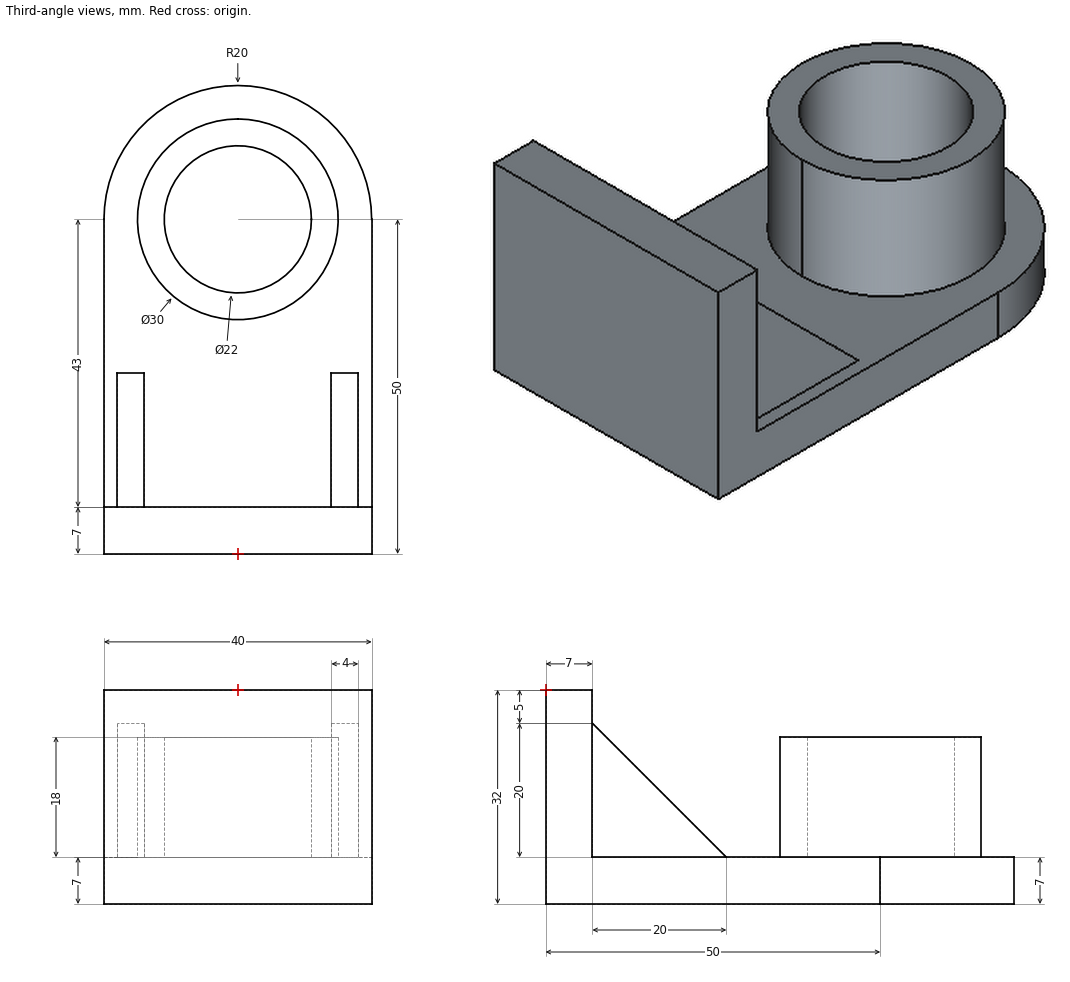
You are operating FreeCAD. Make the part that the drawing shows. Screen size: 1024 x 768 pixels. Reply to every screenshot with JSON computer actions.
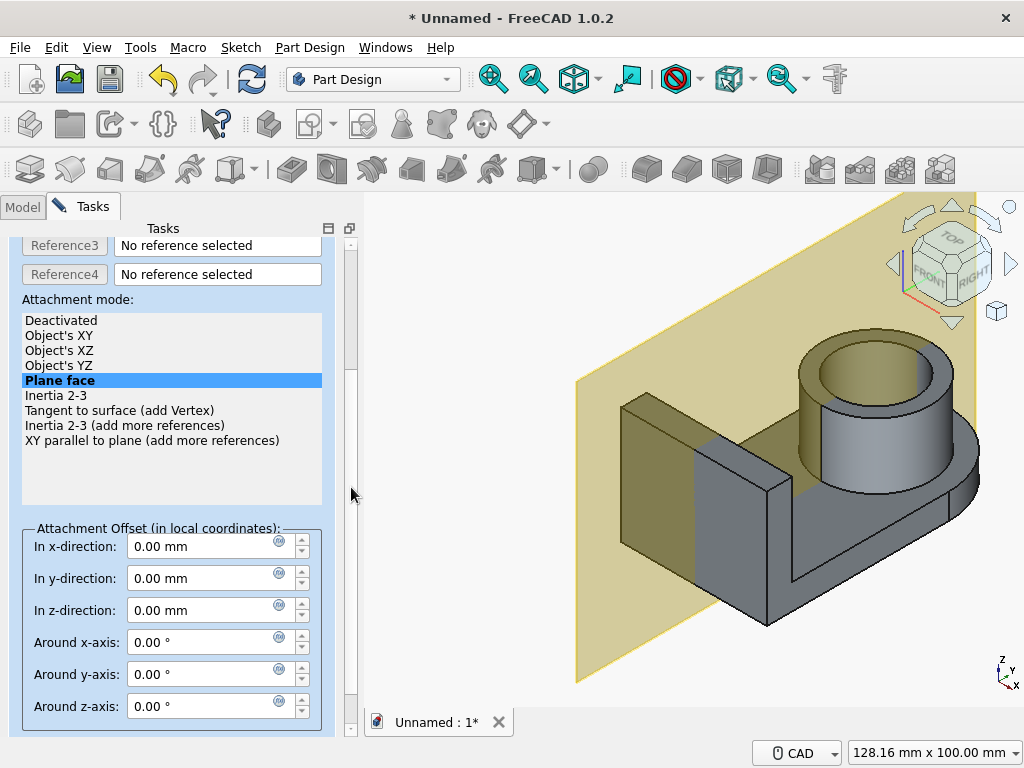
{"action": "triple_click", "coordinate": [210, 610]}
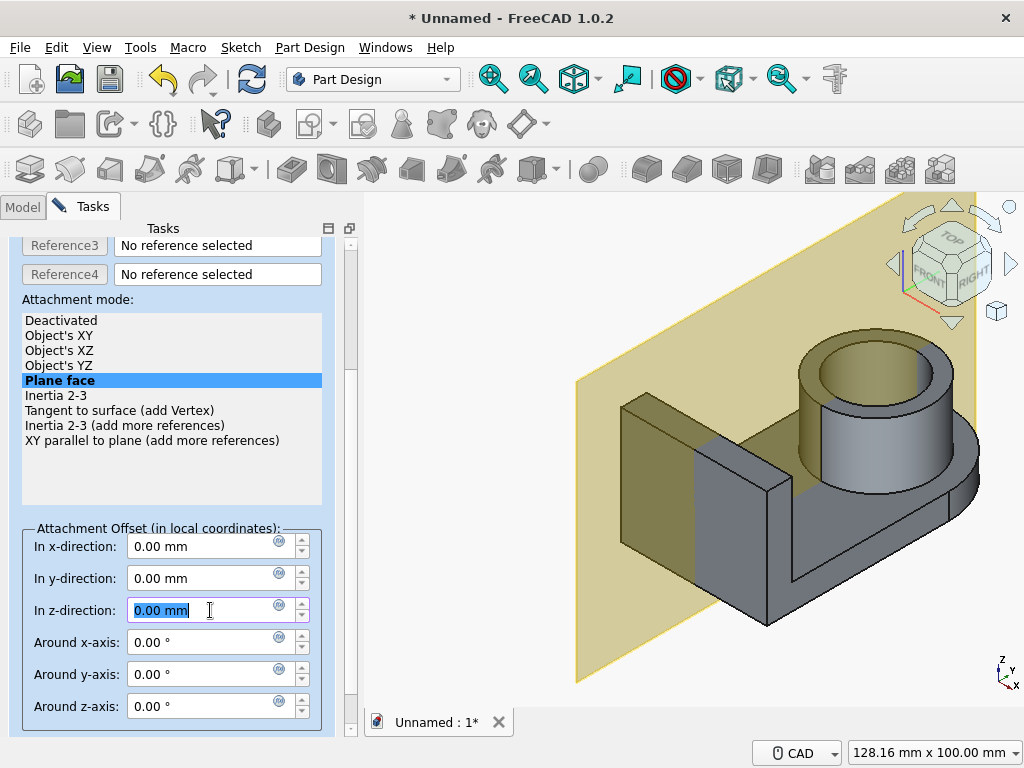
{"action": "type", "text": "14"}
{"action": "key", "text": "Tab"}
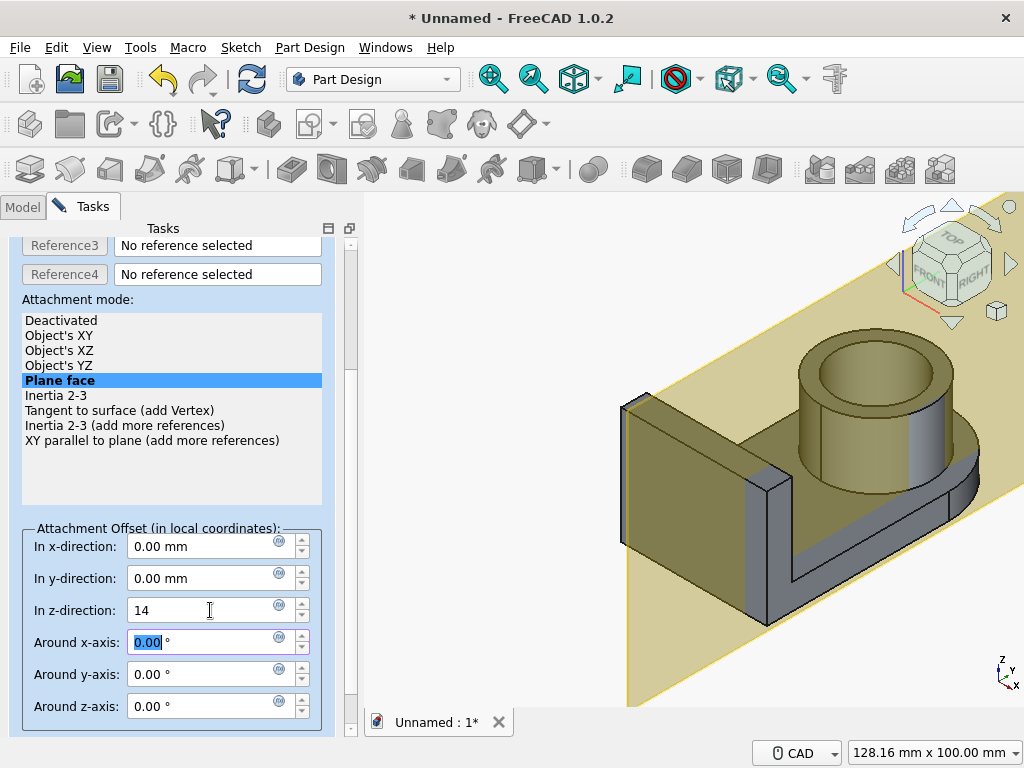
{"action": "scroll", "coordinate": [351, 487], "scroll_direction": "up", "scroll_amount": 4}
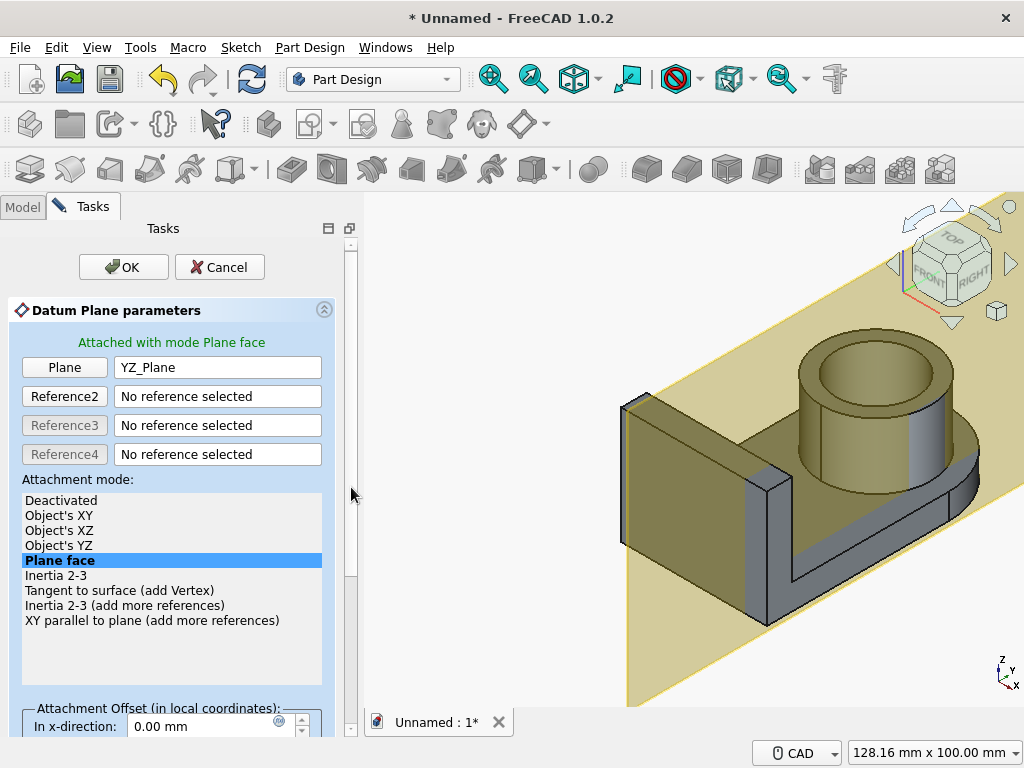
{"action": "left_click", "coordinate": [124, 267]}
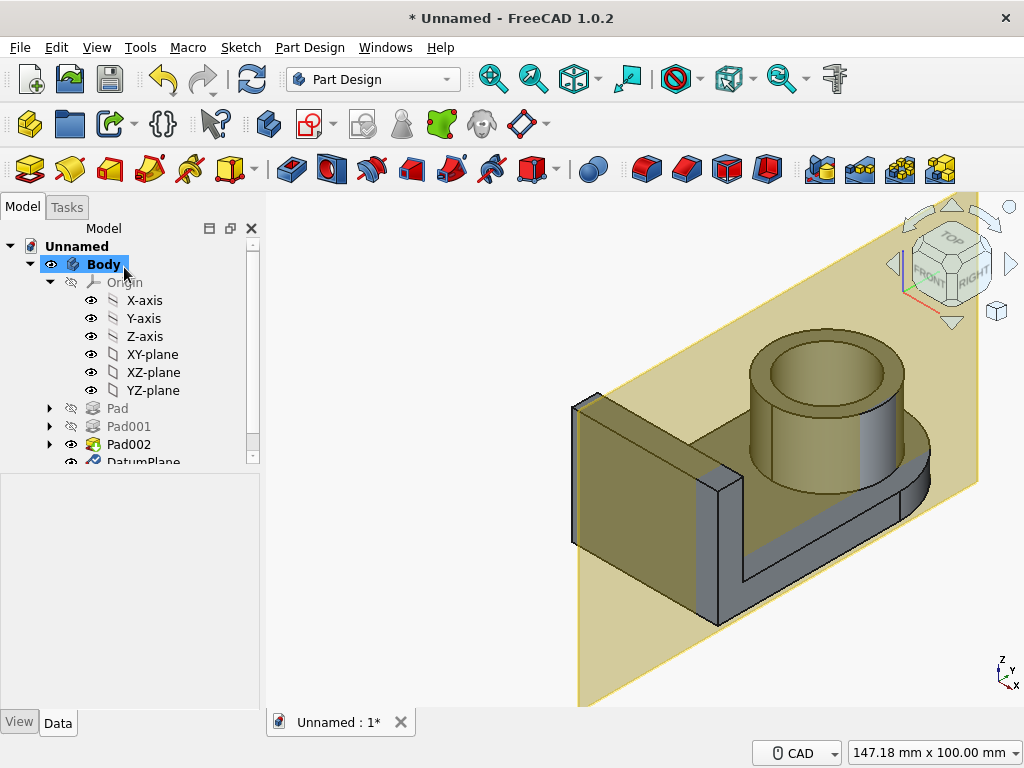
{"action": "left_click", "coordinate": [116, 462]}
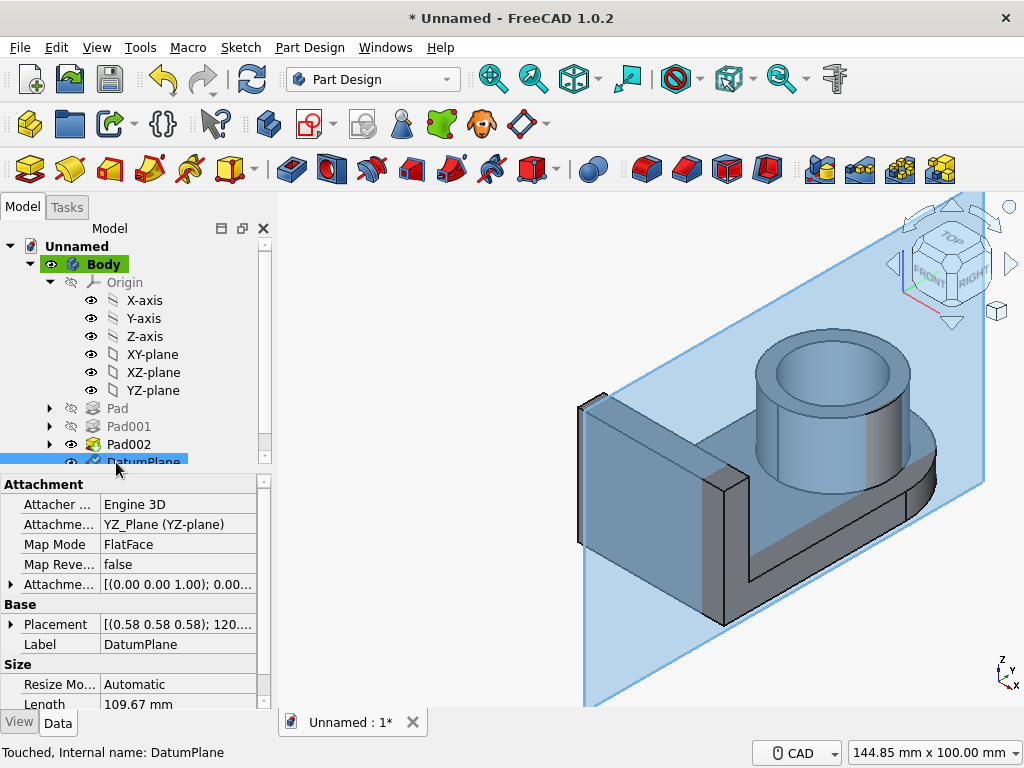
{"action": "left_click", "coordinate": [310, 124]}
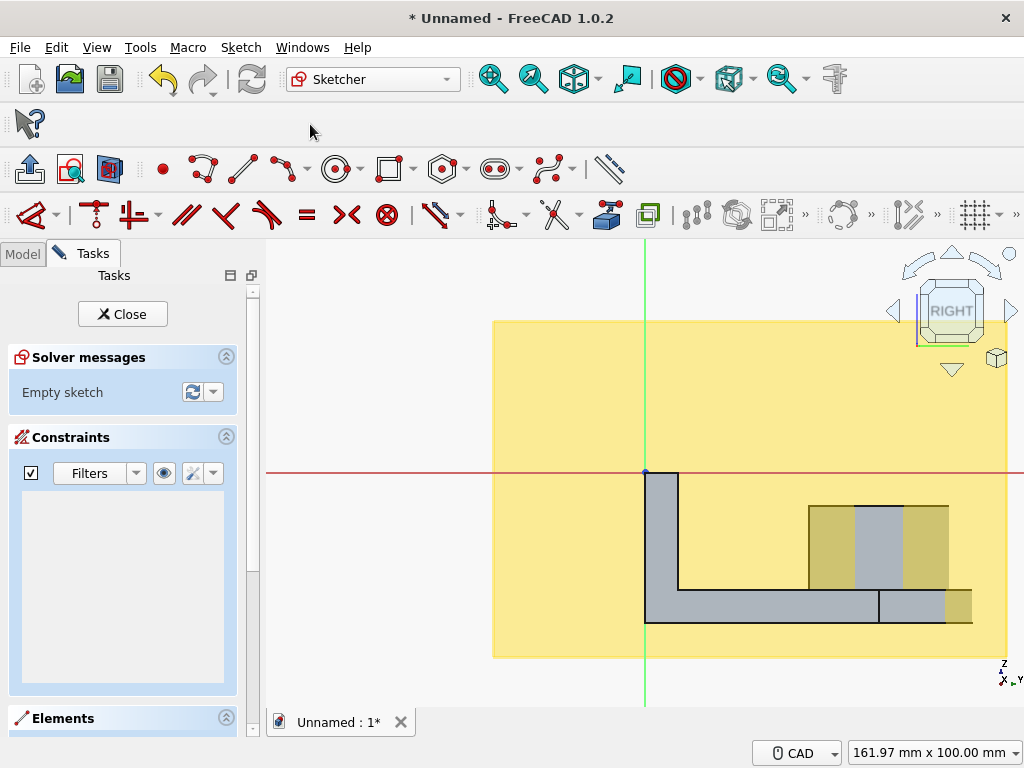
{"action": "left_click", "coordinate": [110, 170]}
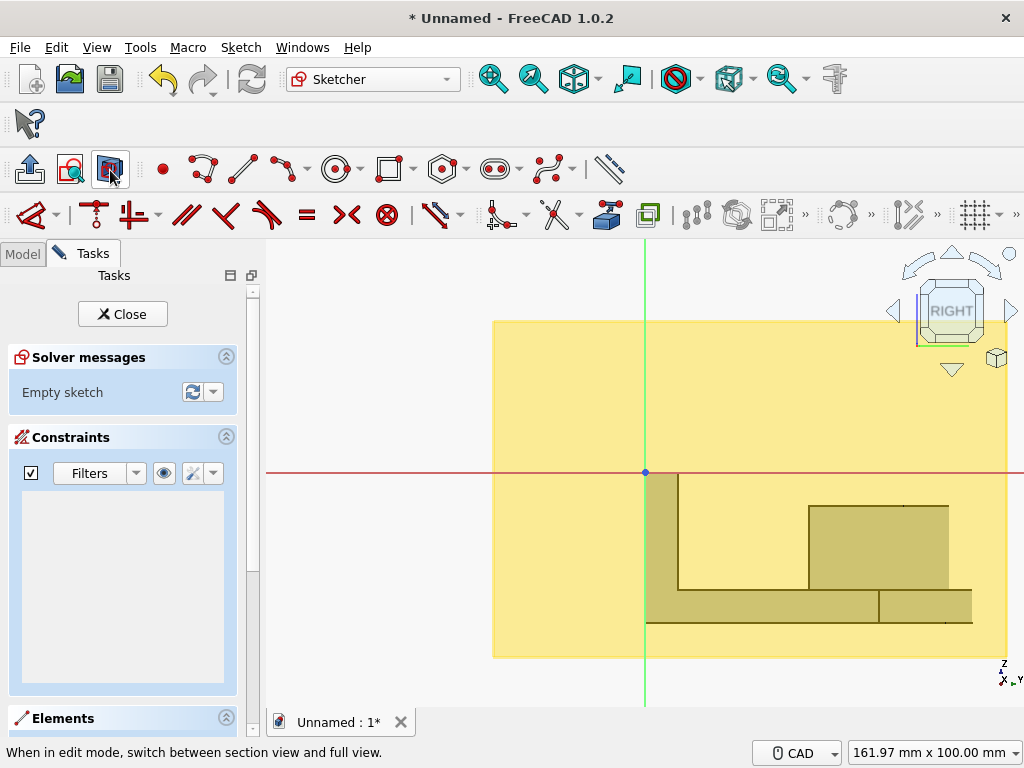
{"action": "scroll", "coordinate": [785, 566], "scroll_direction": "up", "scroll_amount": 5}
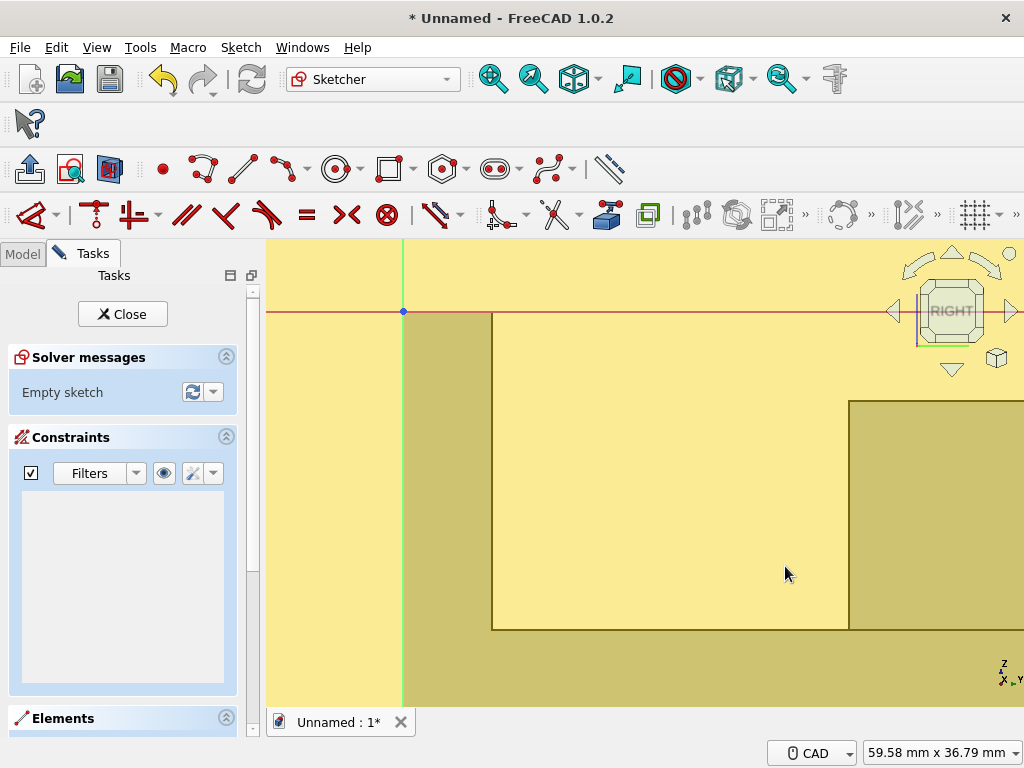
{"action": "left_click", "coordinate": [204, 170]}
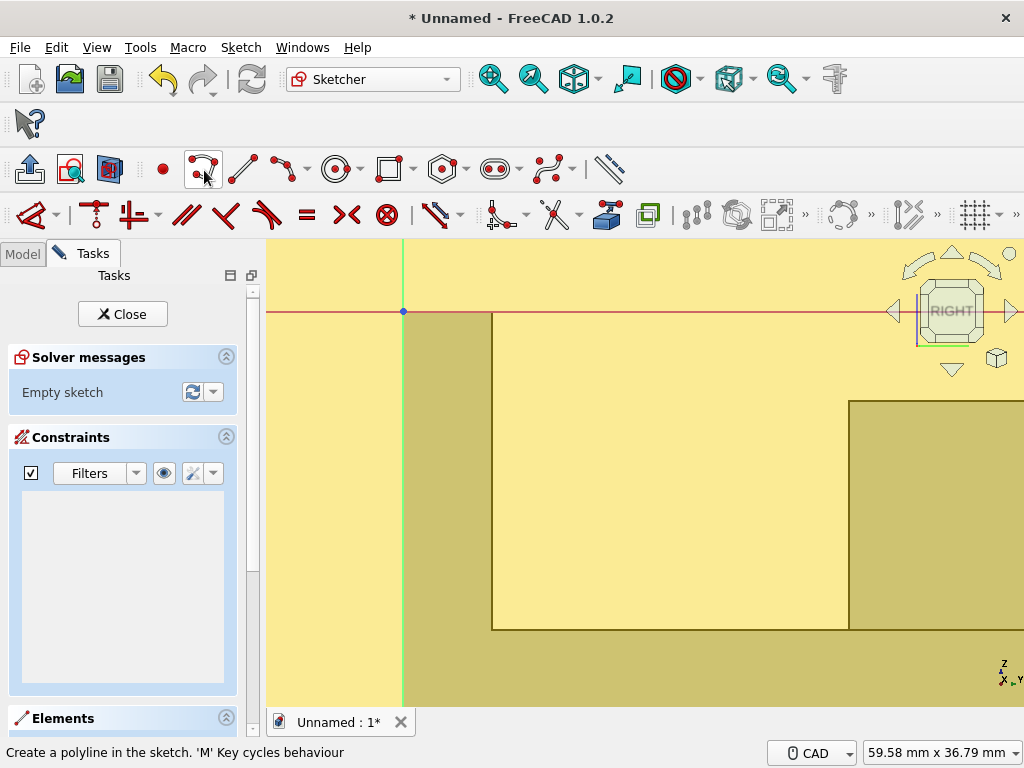
{"action": "left_click", "coordinate": [492, 376]}
{"action": "left_click", "coordinate": [492, 630]}
{"action": "left_click", "coordinate": [747, 630]}
{"action": "left_click", "coordinate": [492, 377]}
{"action": "key", "text": "Escape"}
{"action": "key", "text": "Escape"}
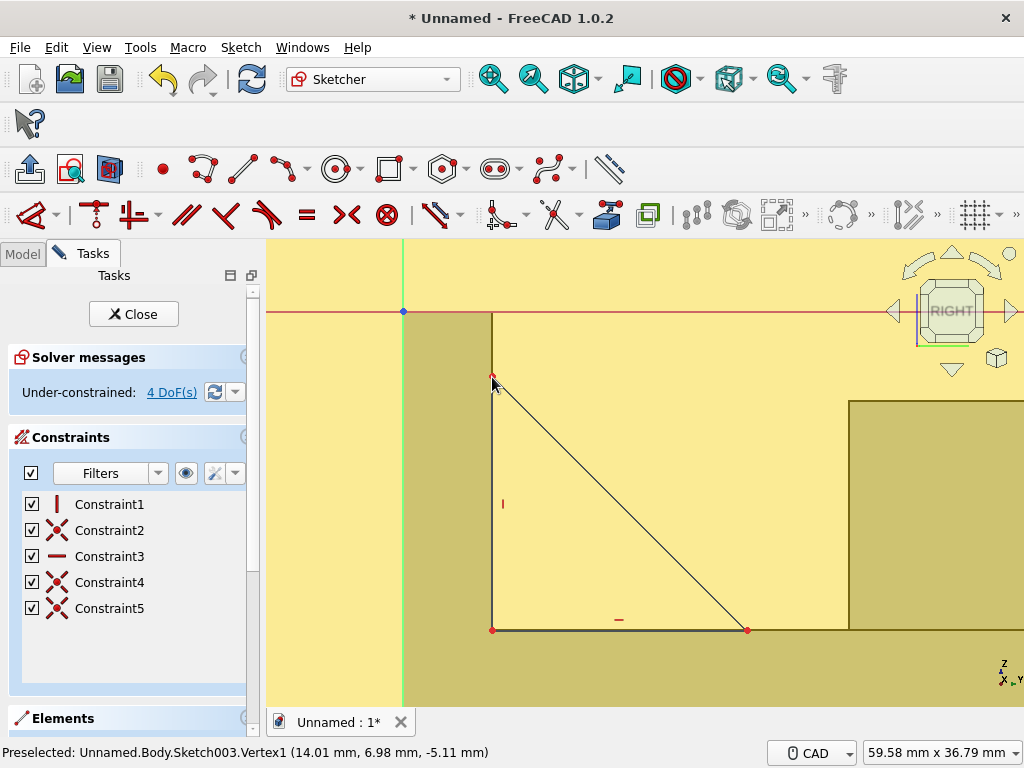
{"action": "left_click", "coordinate": [32, 216]}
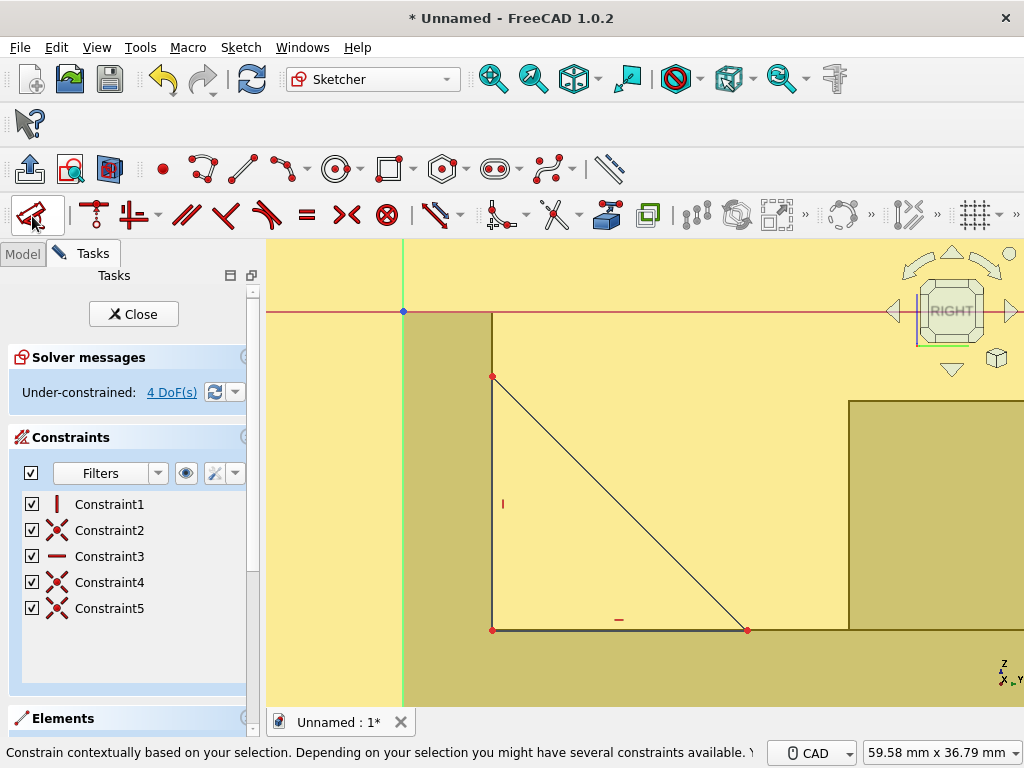
{"action": "left_click", "coordinate": [492, 453]}
{"action": "left_click", "coordinate": [458, 504]}